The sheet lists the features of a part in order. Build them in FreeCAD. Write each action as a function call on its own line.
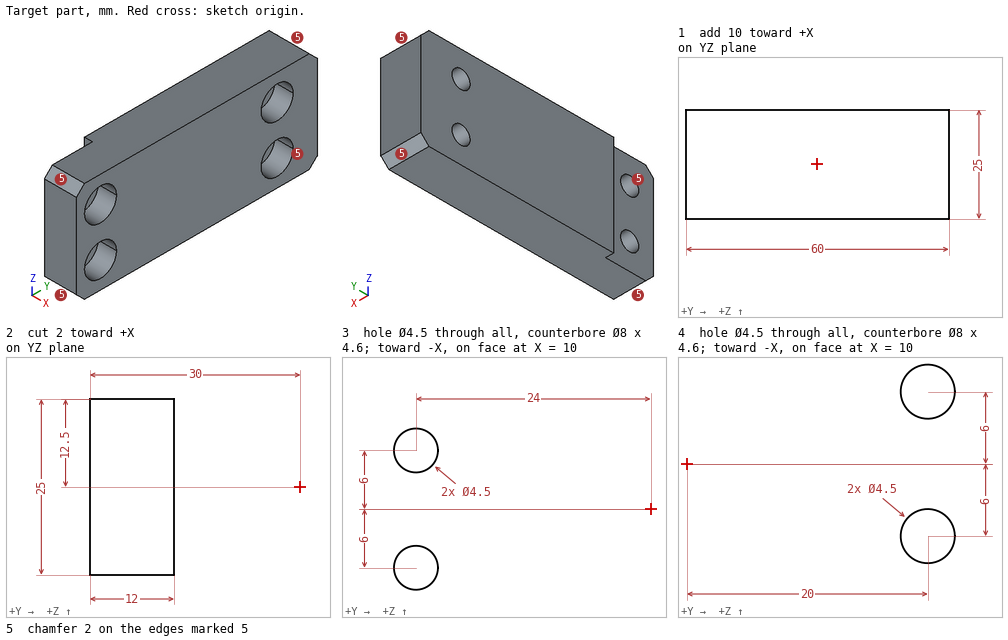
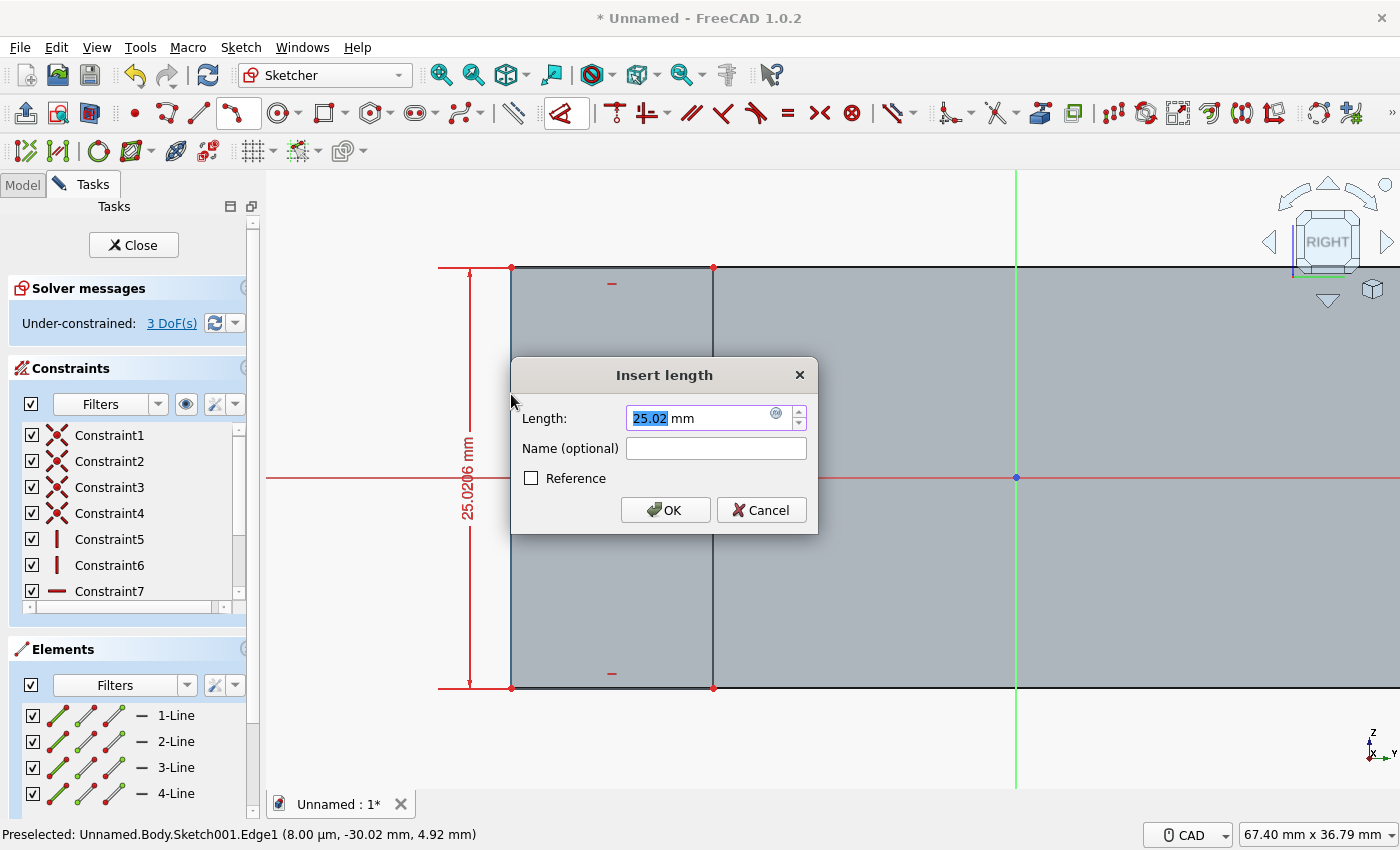
text(25)
key(Return)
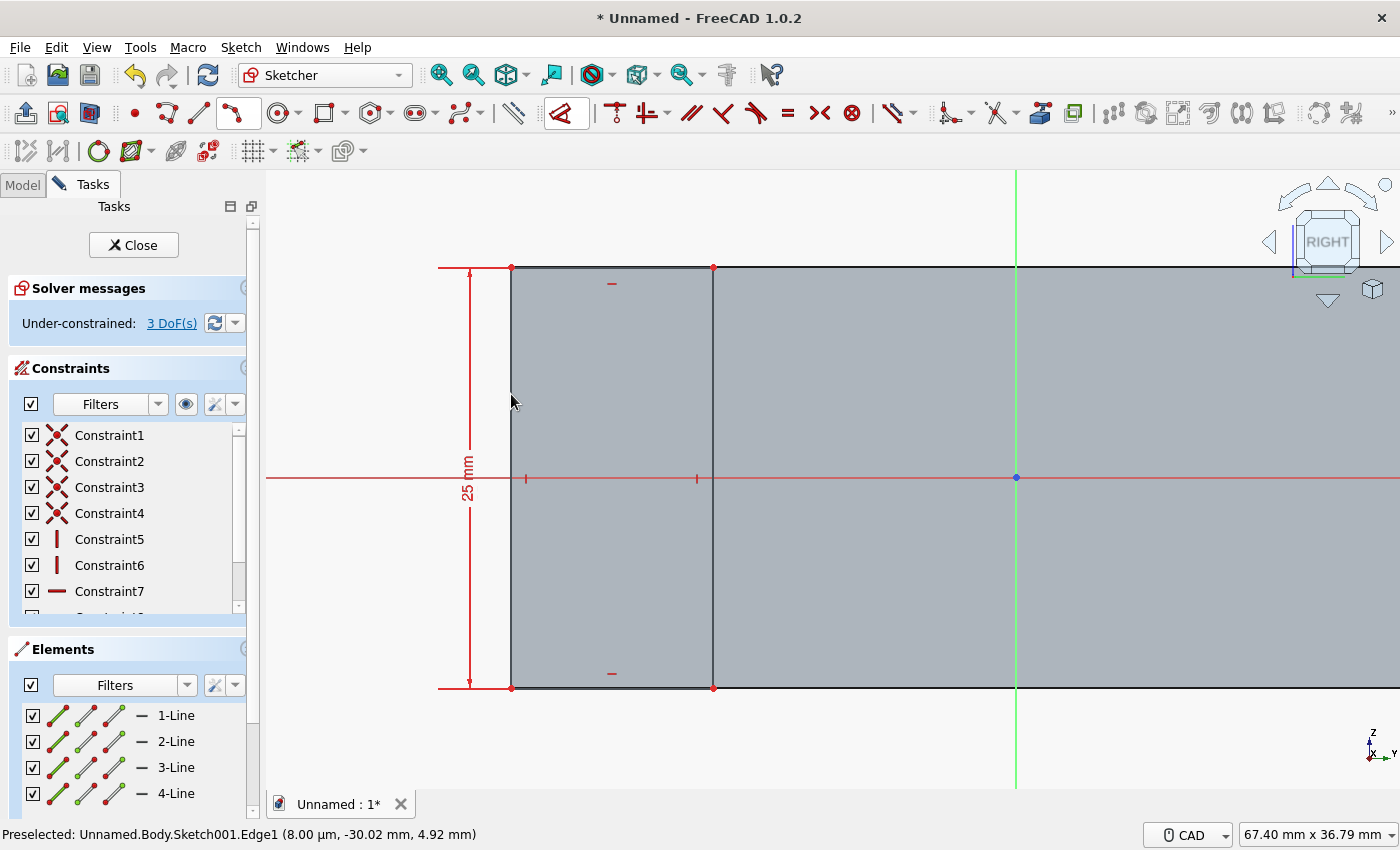
click(572, 689)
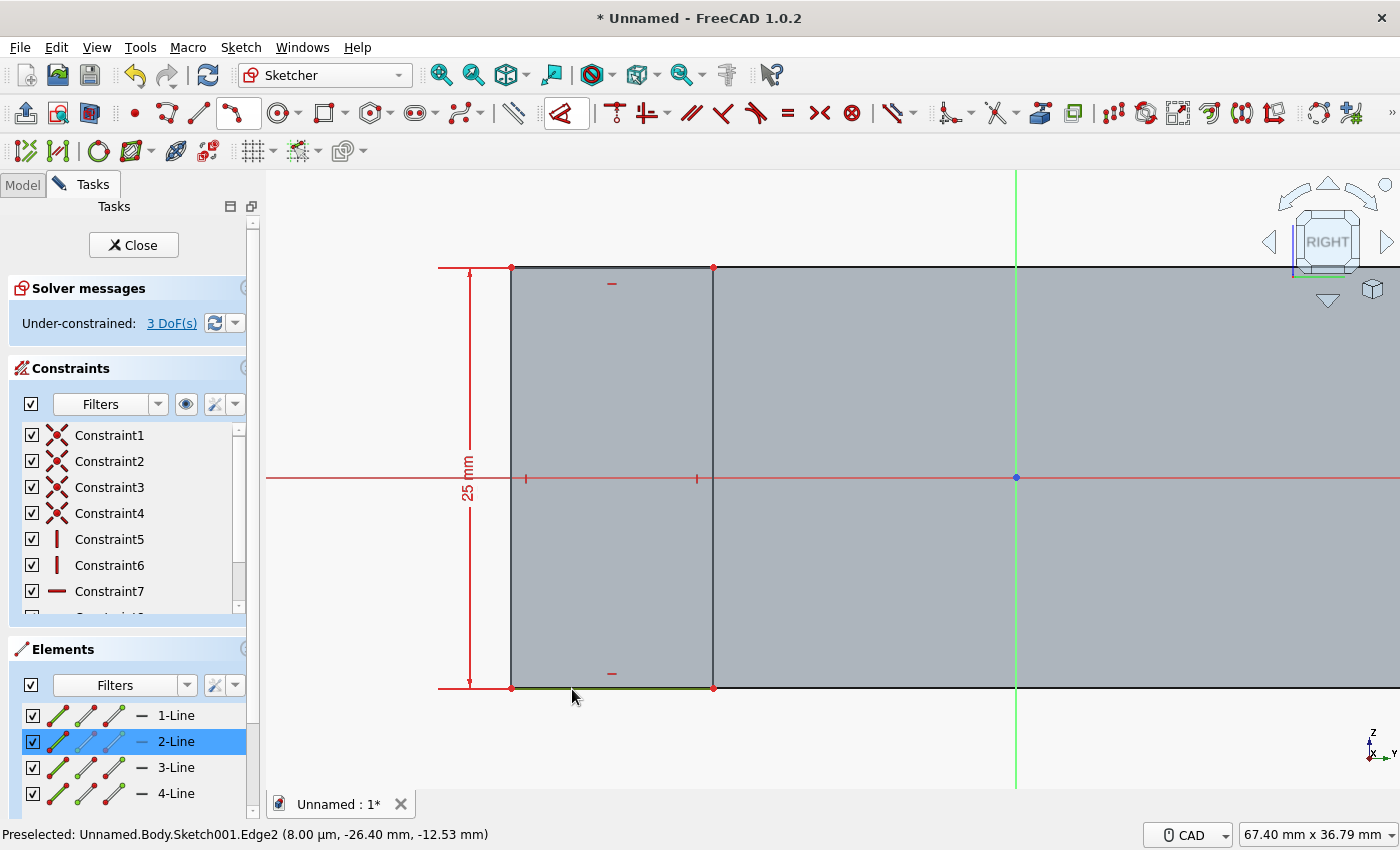
click(584, 114)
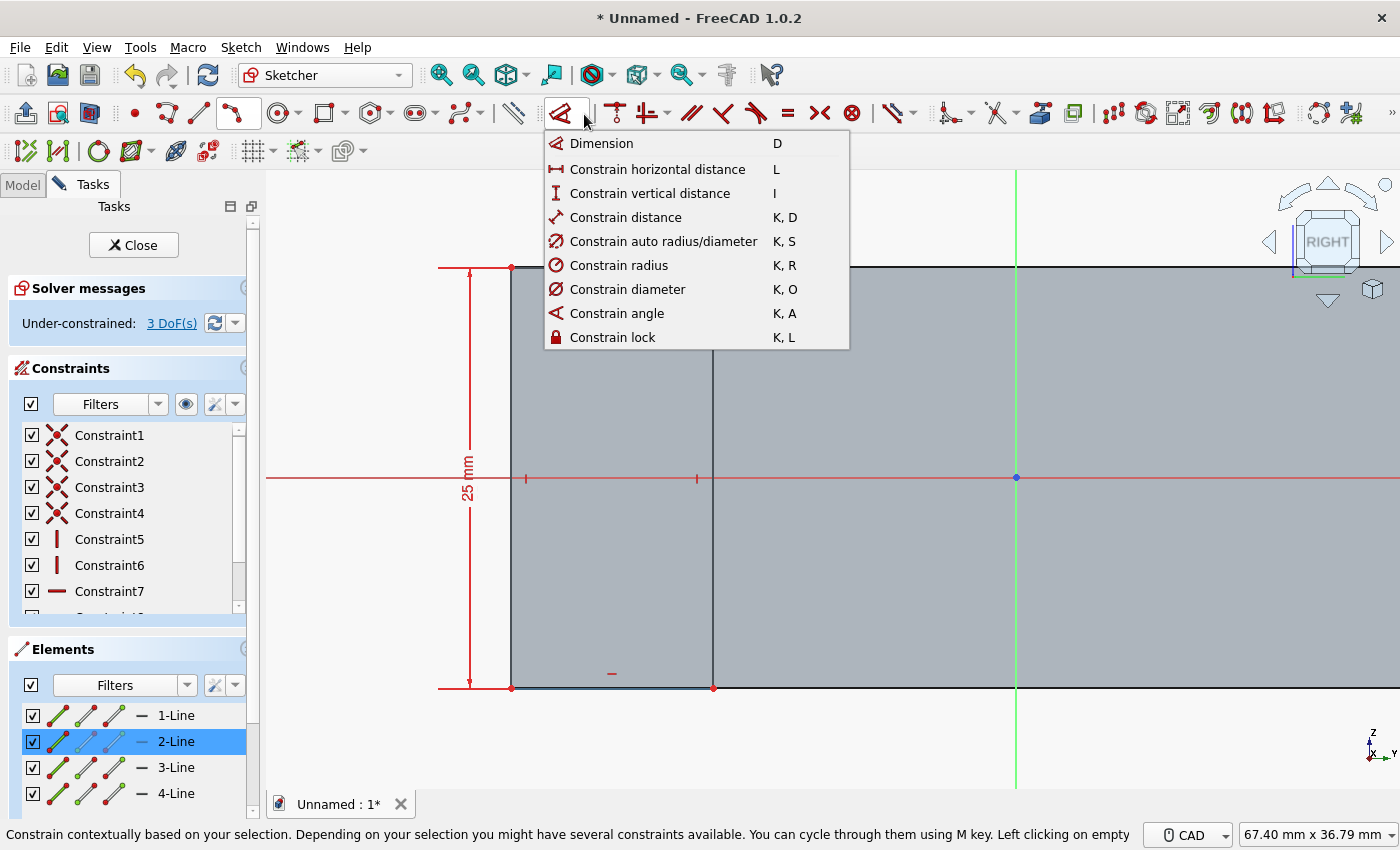
click(697, 169)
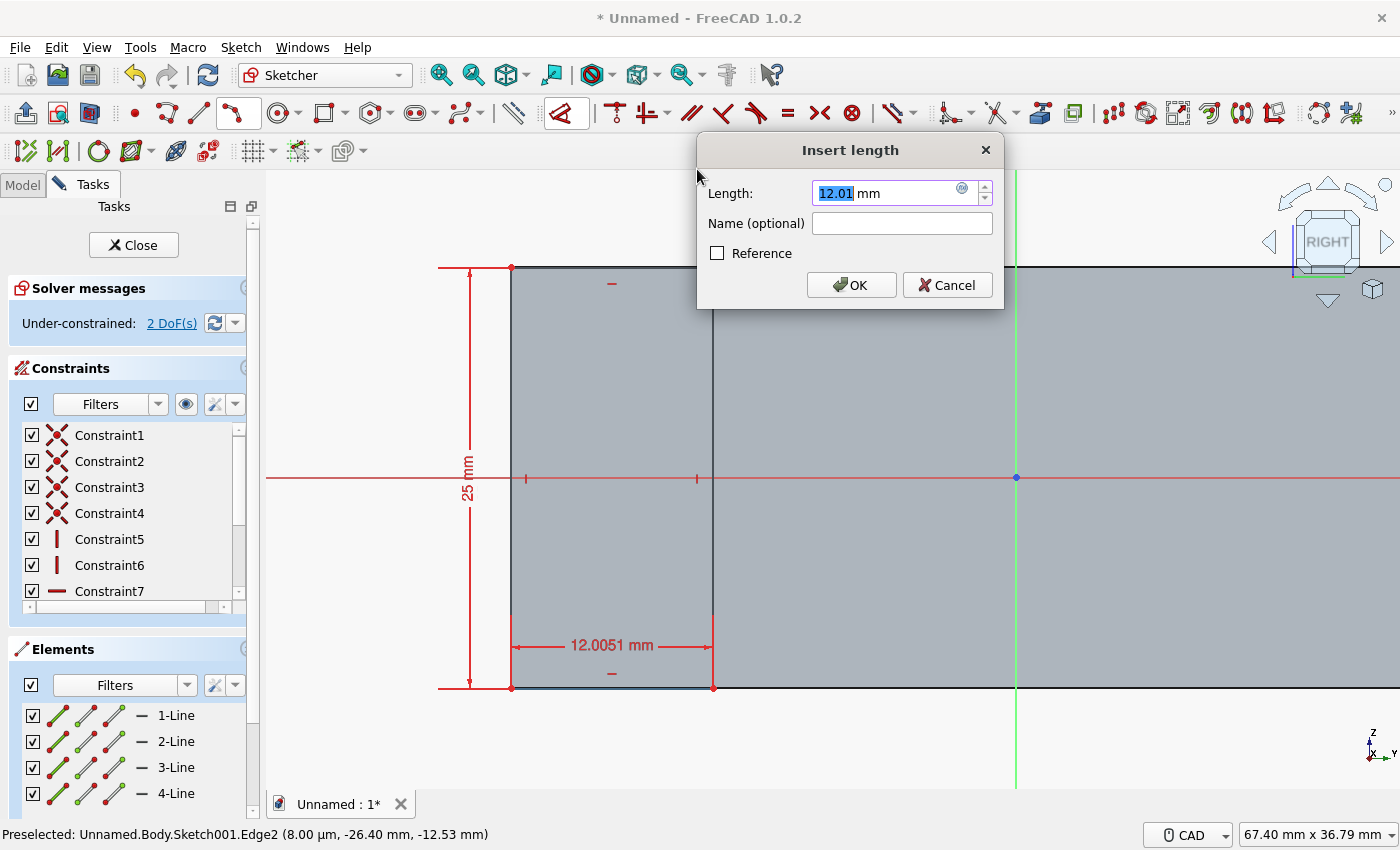
text(12)
key(Return)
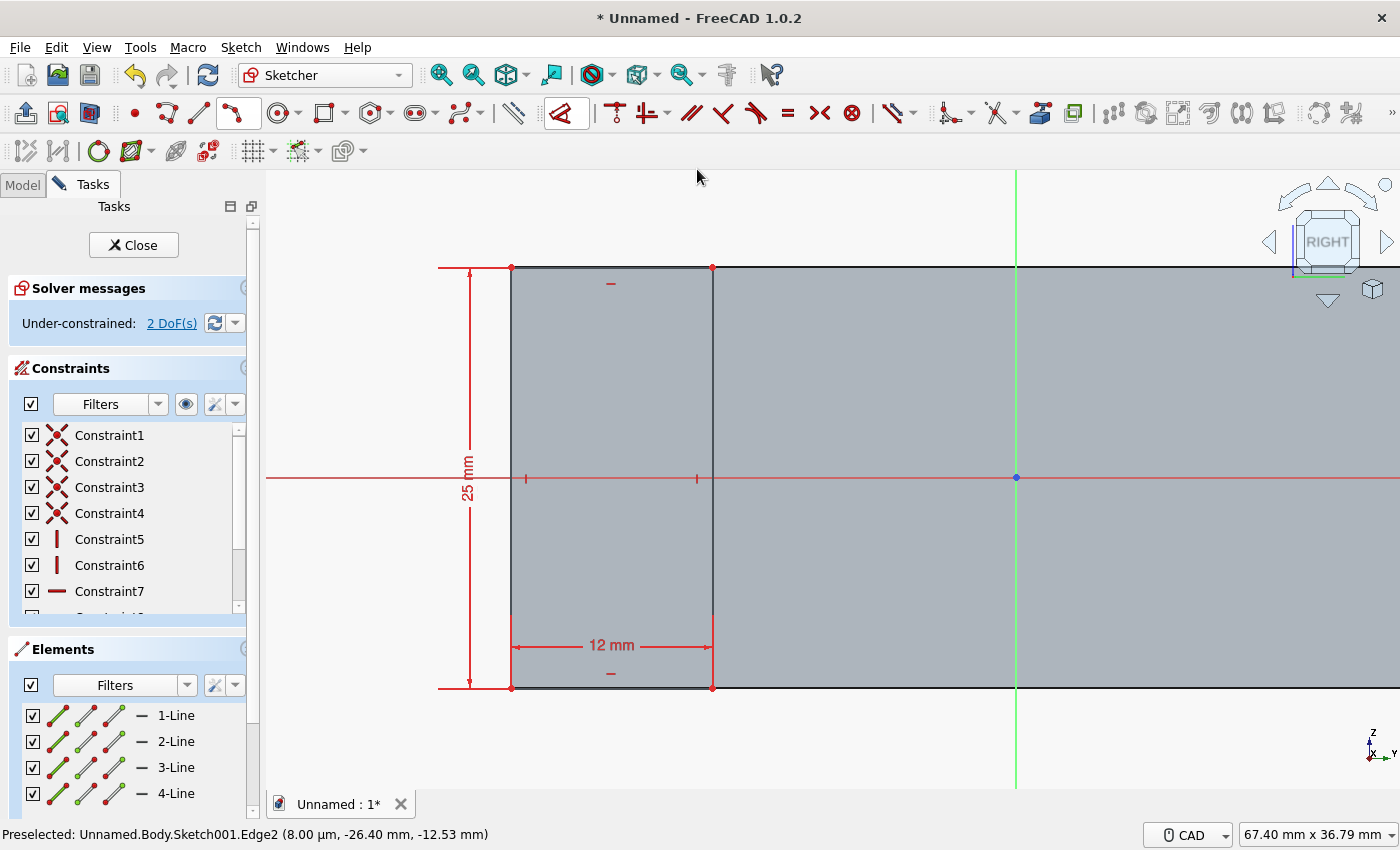
click(511, 268)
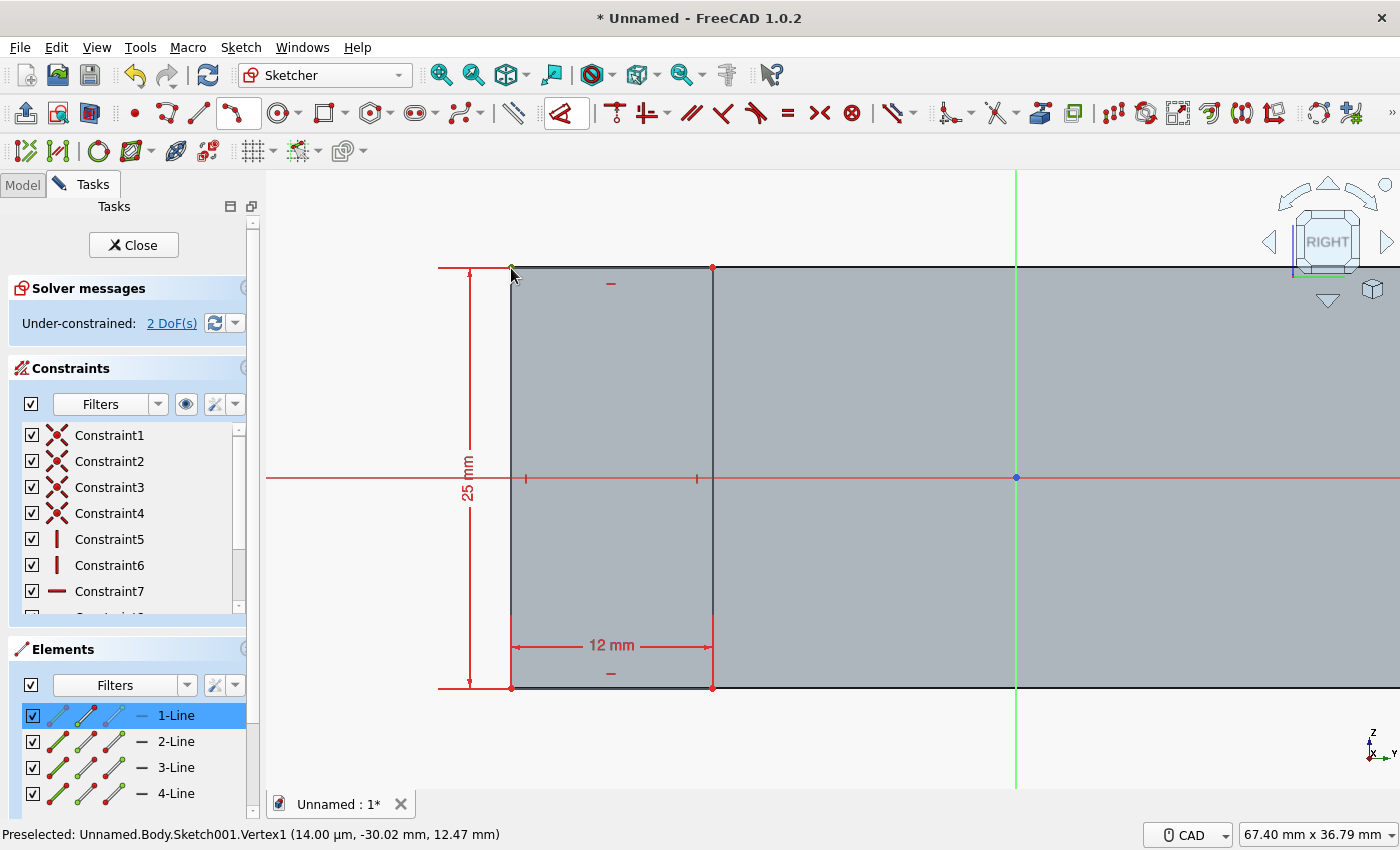
key(l)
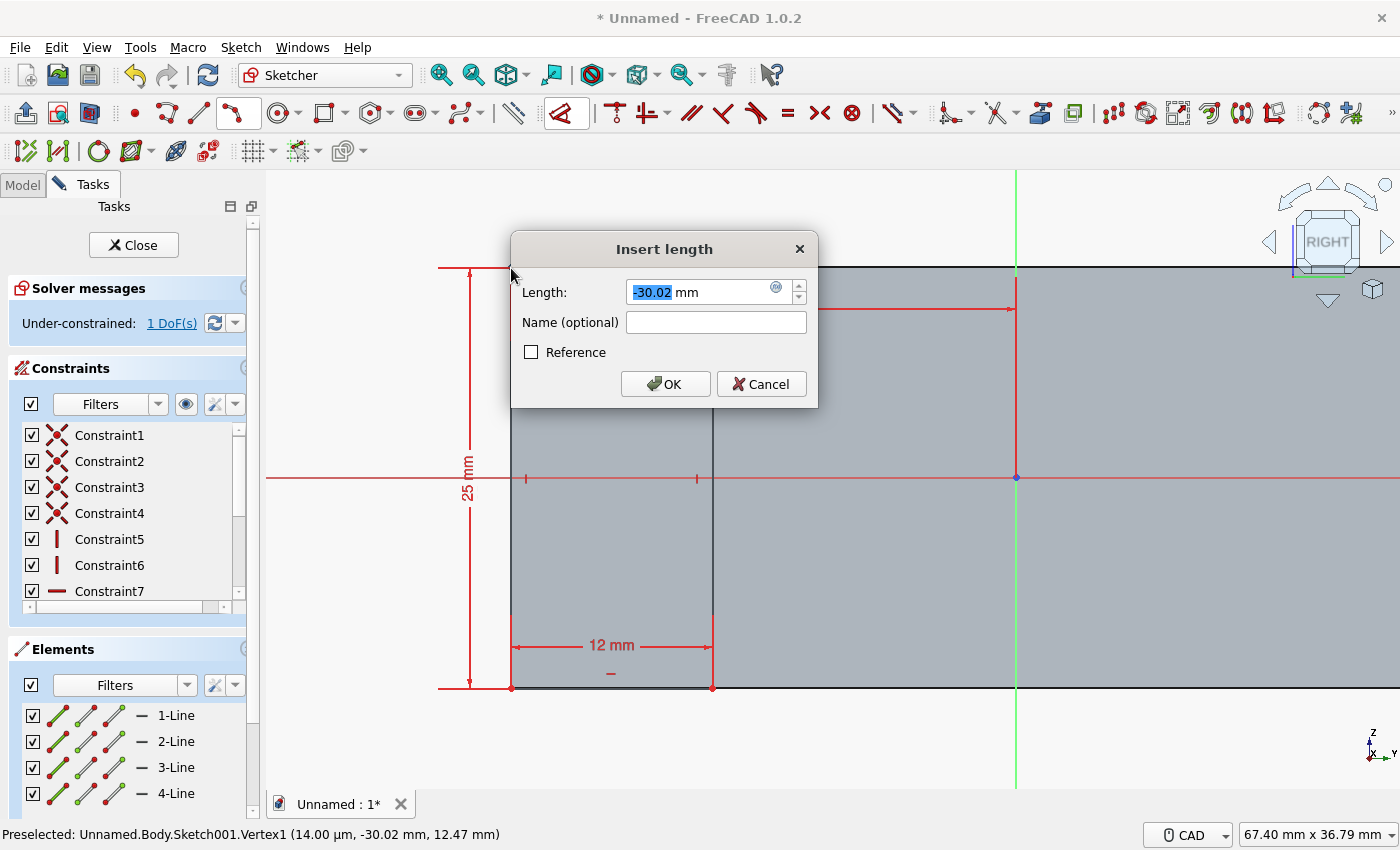
text(-30)
key(Return)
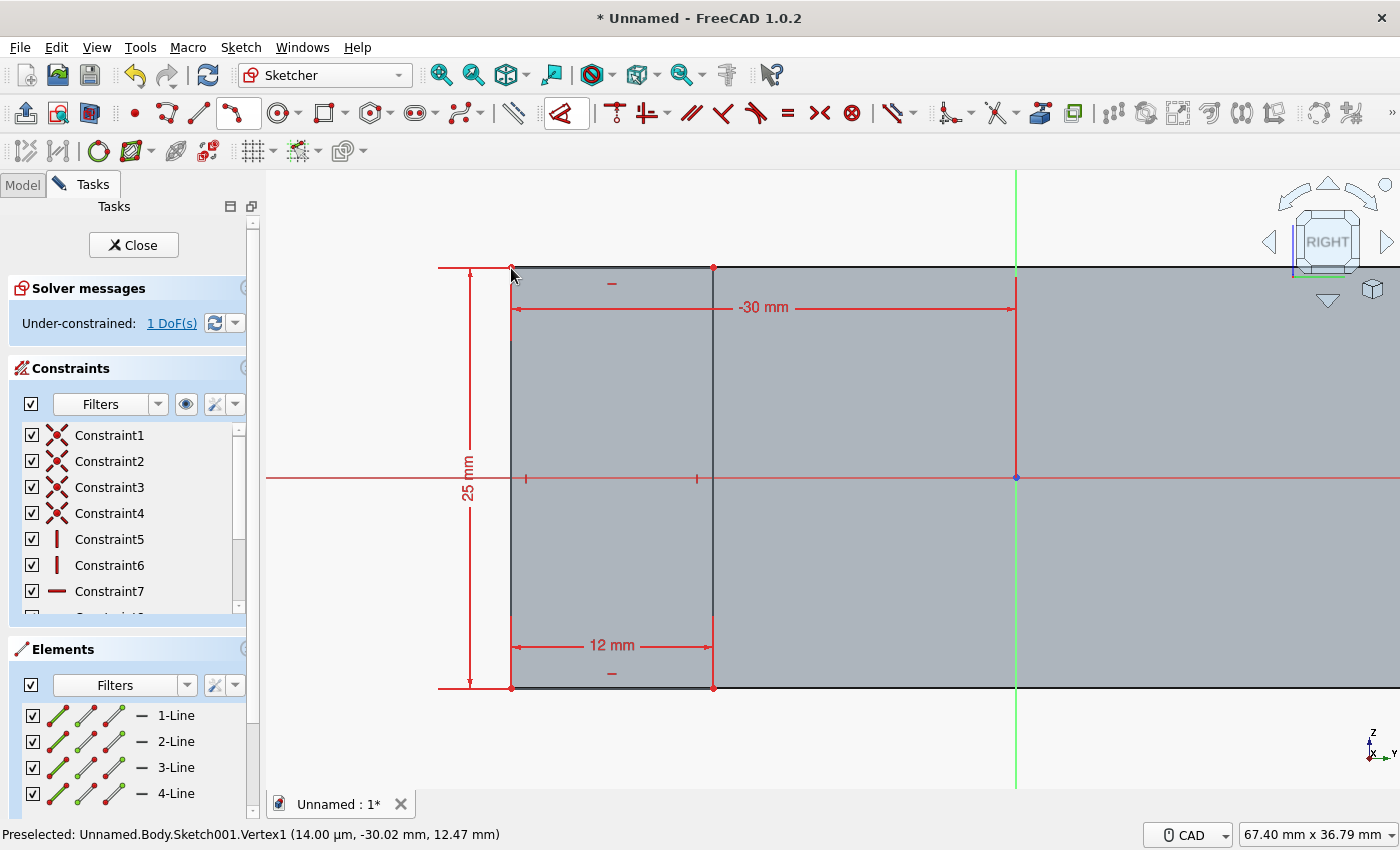
click(511, 268)